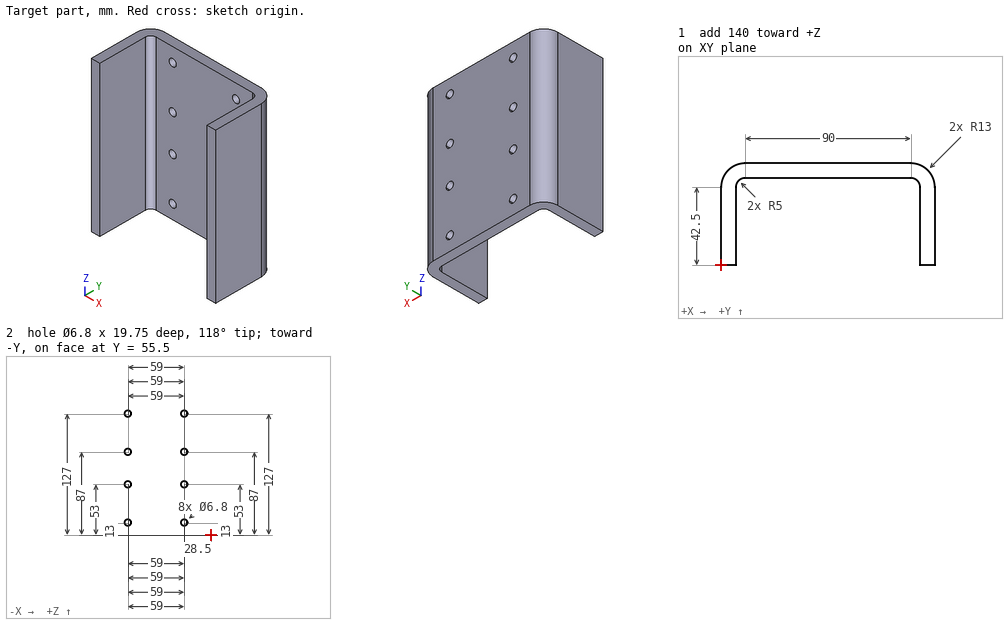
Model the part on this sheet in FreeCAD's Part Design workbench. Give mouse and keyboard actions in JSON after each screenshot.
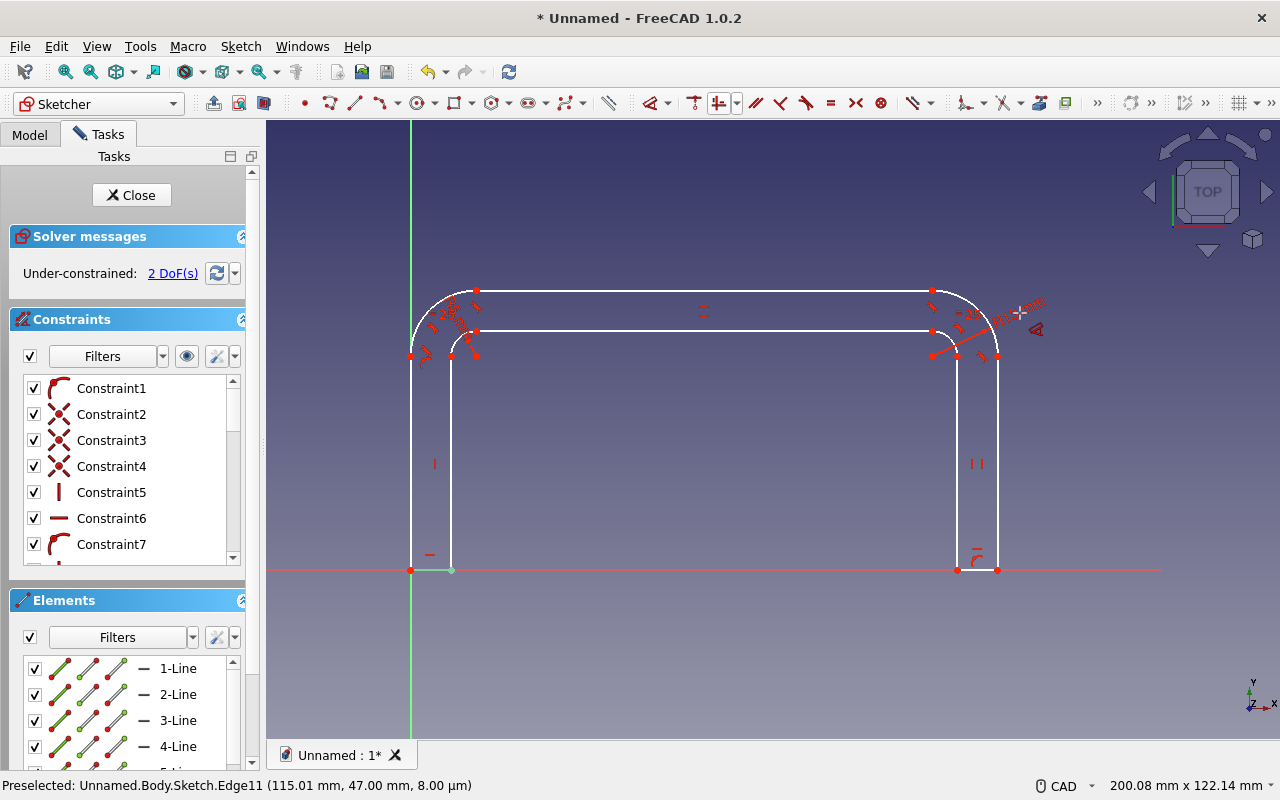
{"action": "left_click", "coordinate": [613, 331]}
{"action": "left_click", "coordinate": [704, 365]}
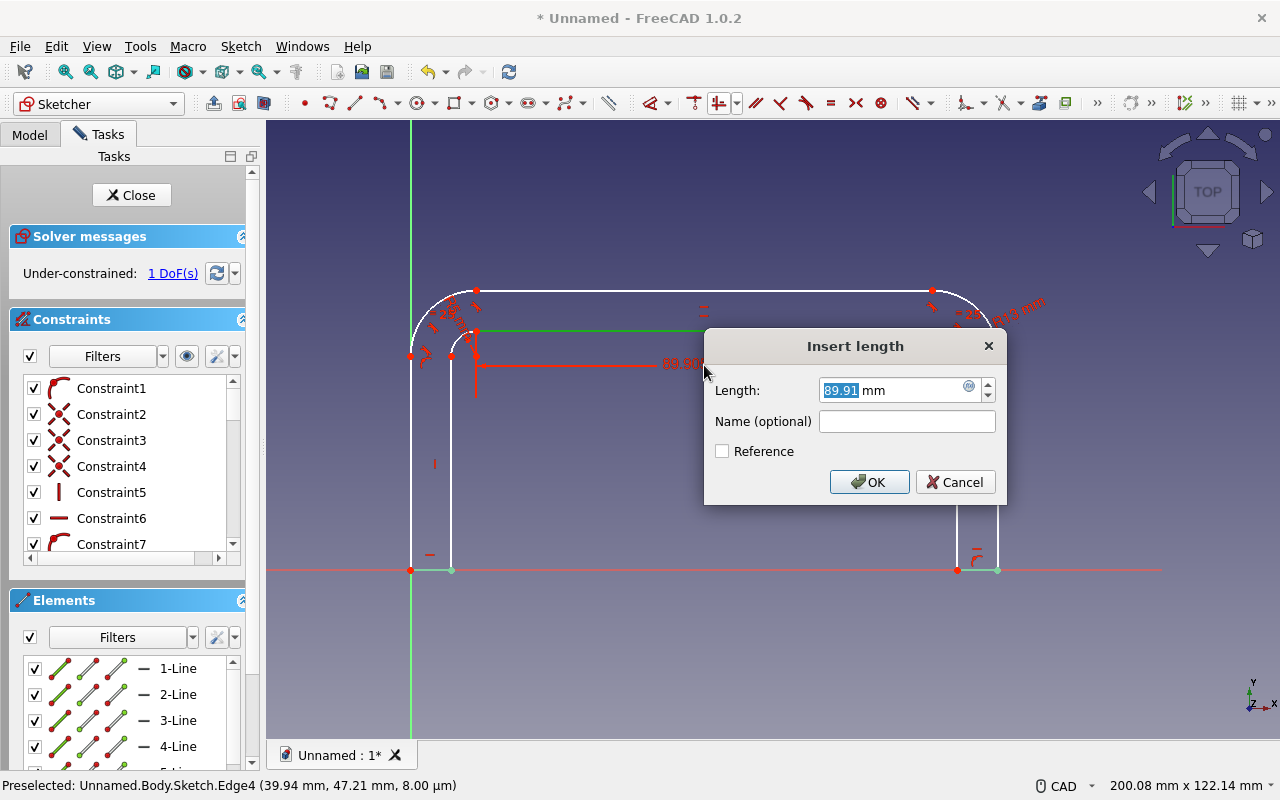
{"action": "type", "text": "90"}
{"action": "key", "text": "Return"}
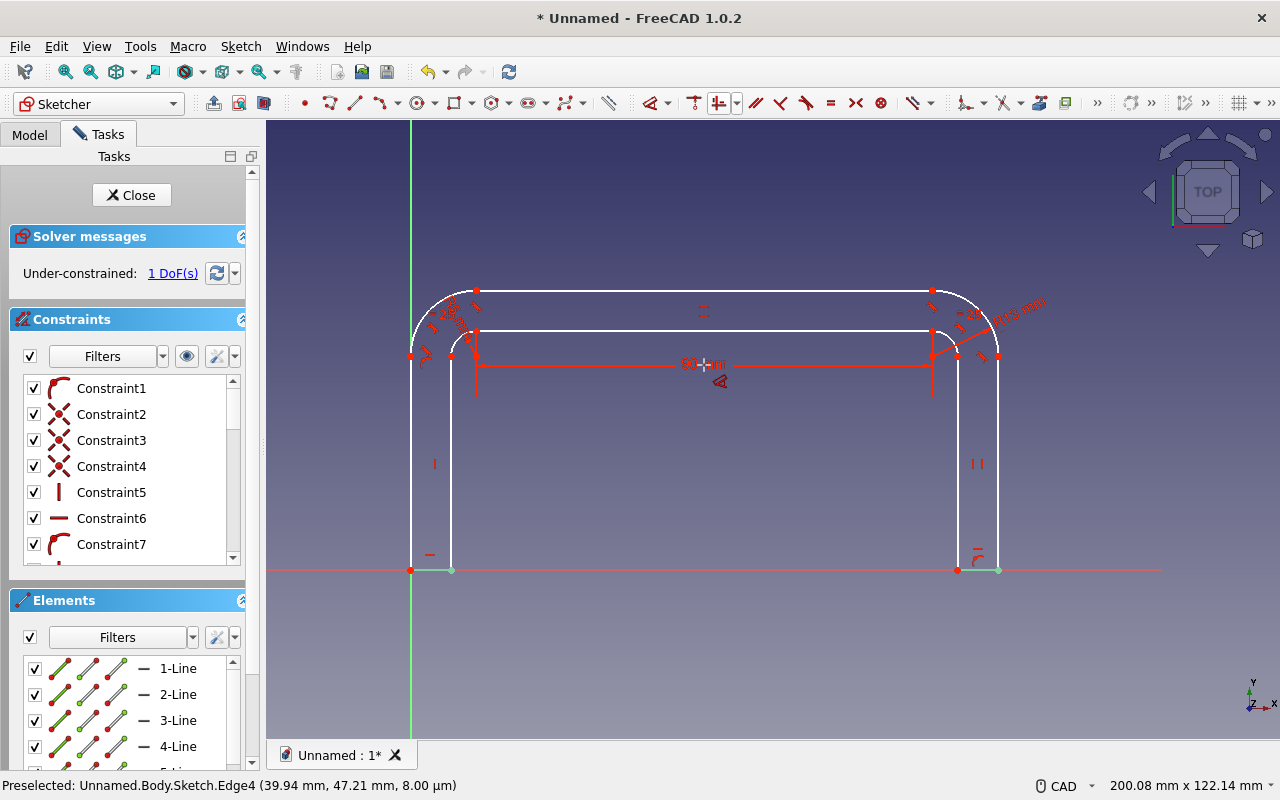
{"action": "left_click", "coordinate": [411, 421]}
{"action": "left_click", "coordinate": [377, 464]}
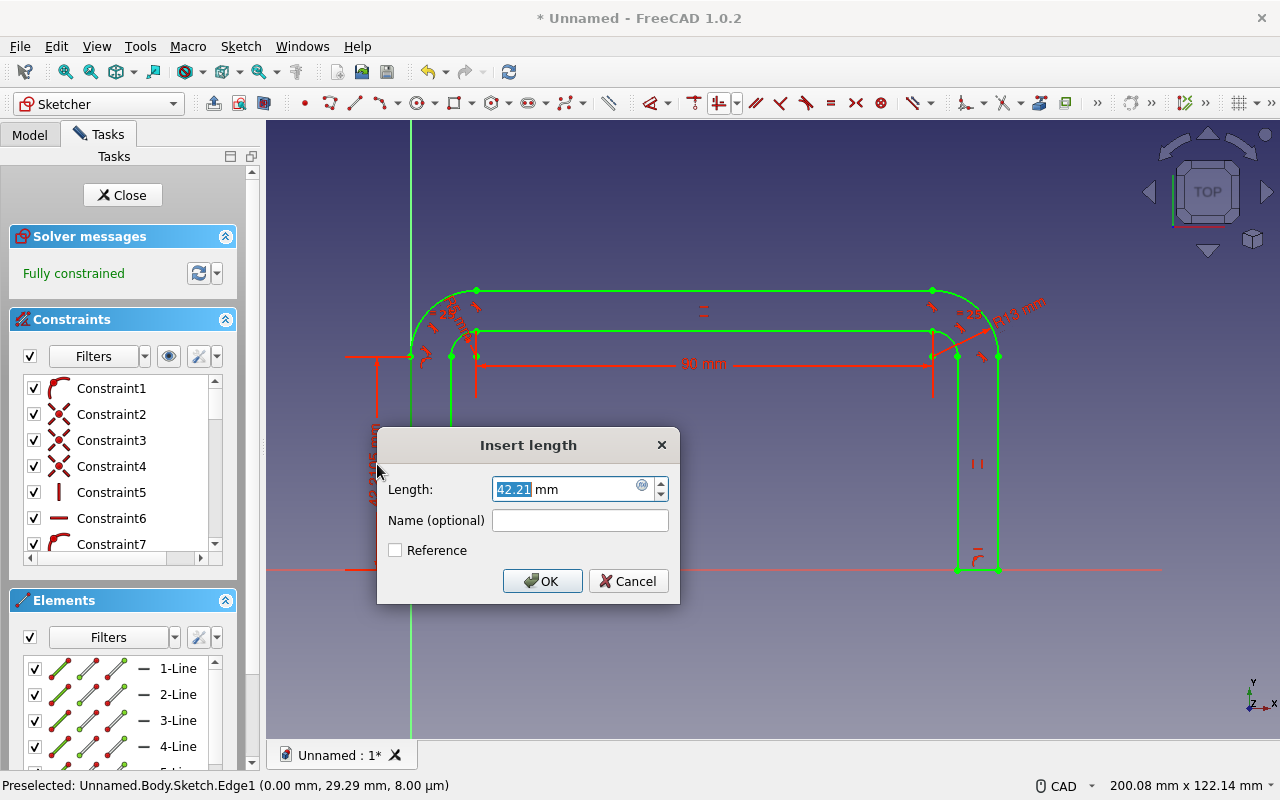
{"action": "type", "text": "42.5"}
{"action": "key", "text": "Return"}
{"action": "key", "text": "Escape"}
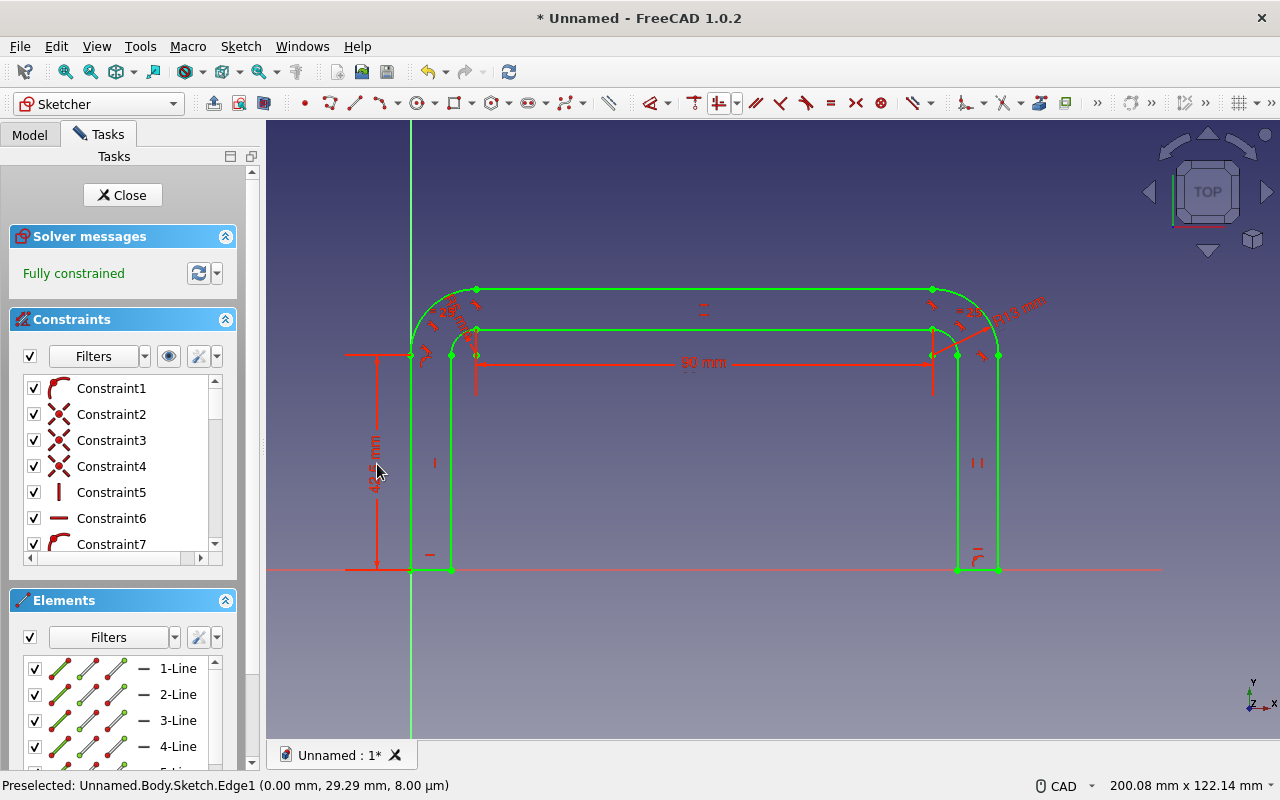
{"action": "left_click", "coordinate": [123, 195]}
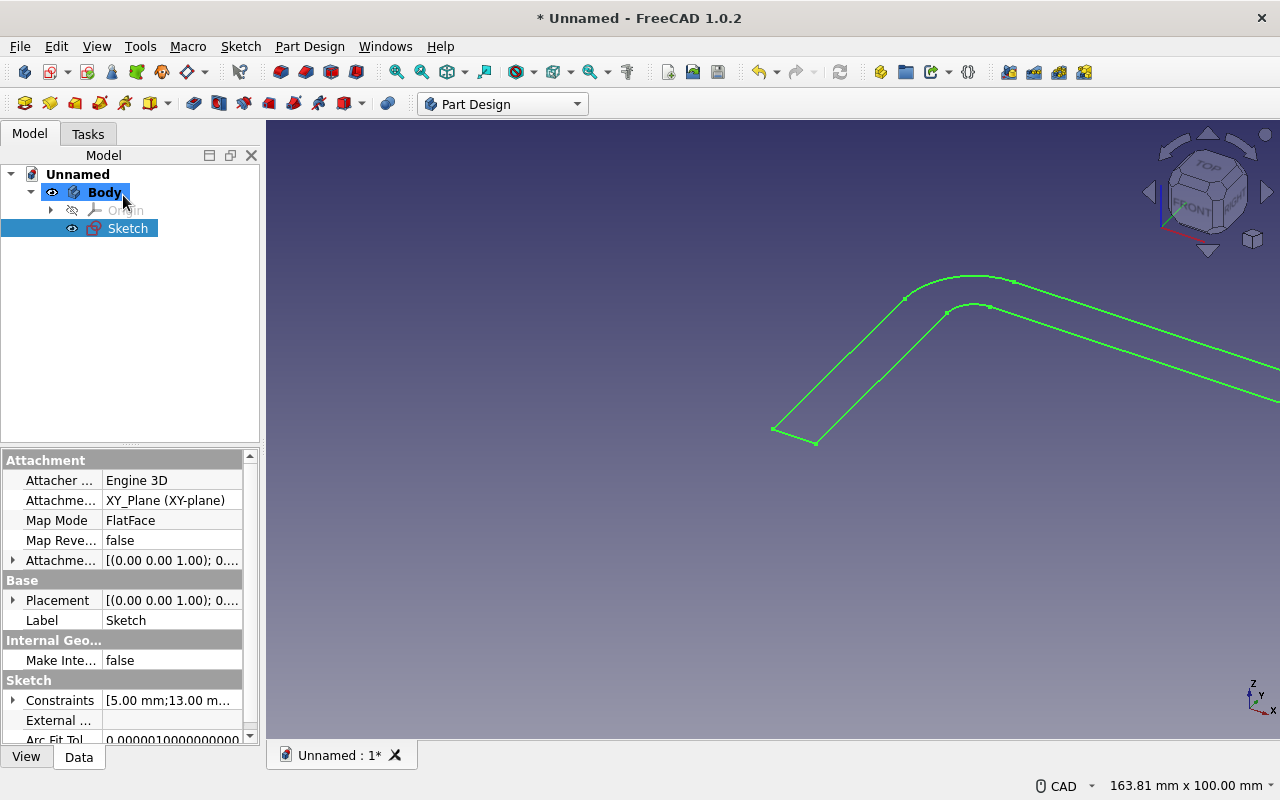
{"action": "left_click", "coordinate": [25, 104]}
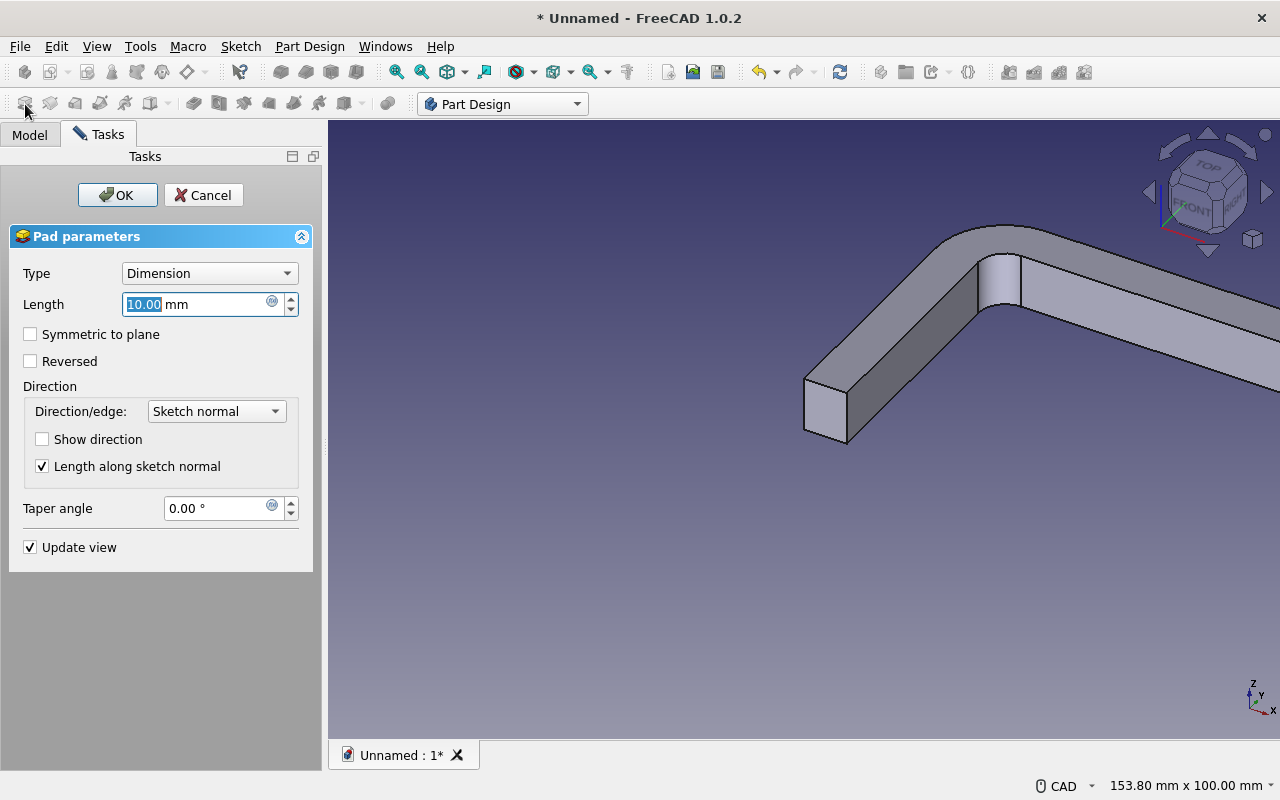
{"action": "type", "text": "140"}
{"action": "key", "text": "Tab"}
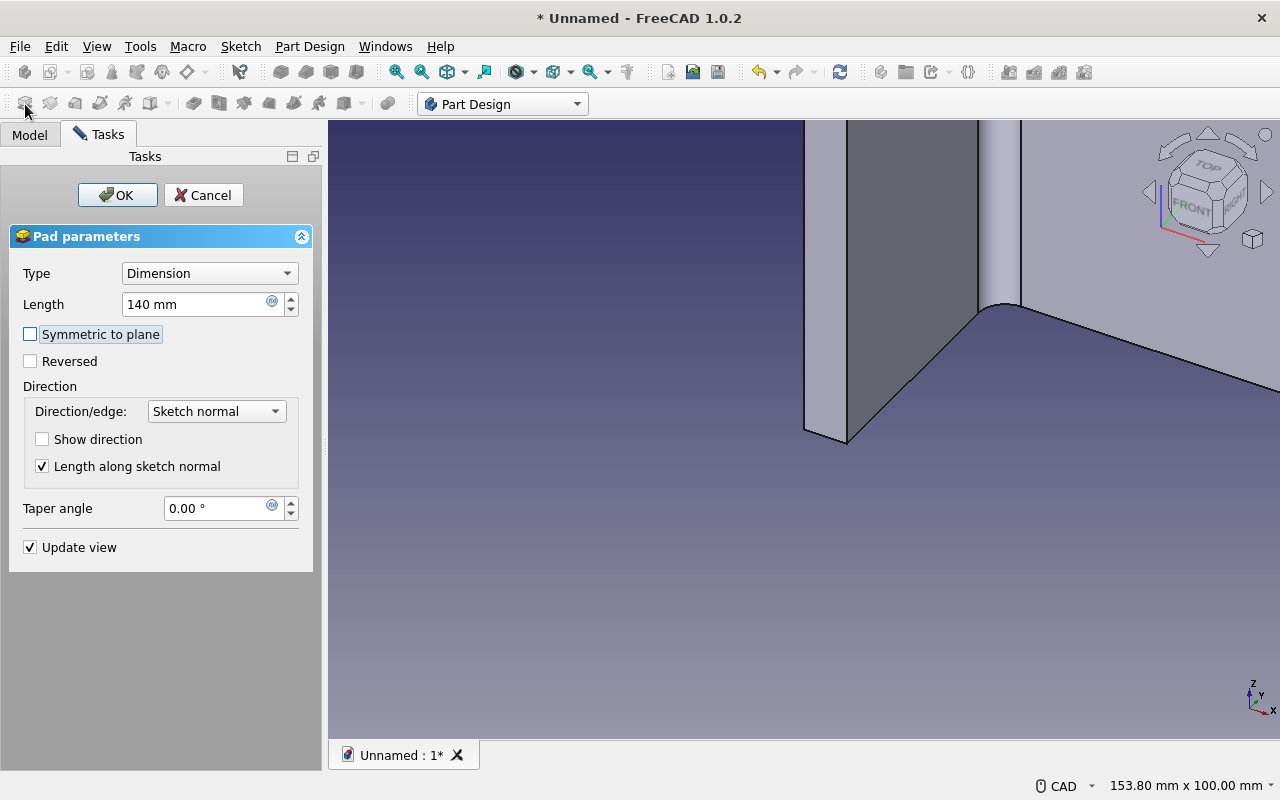
{"action": "left_click", "coordinate": [118, 195]}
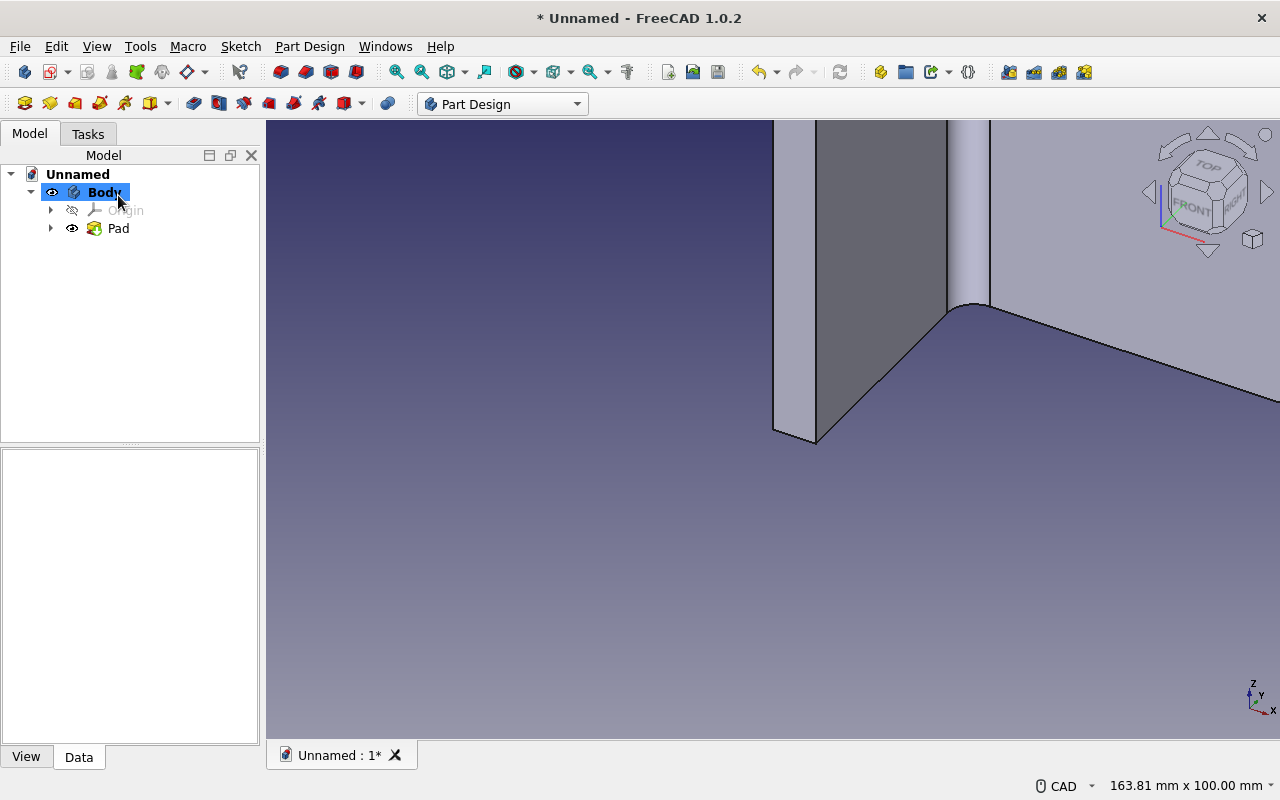
{"action": "left_click", "coordinate": [397, 72]}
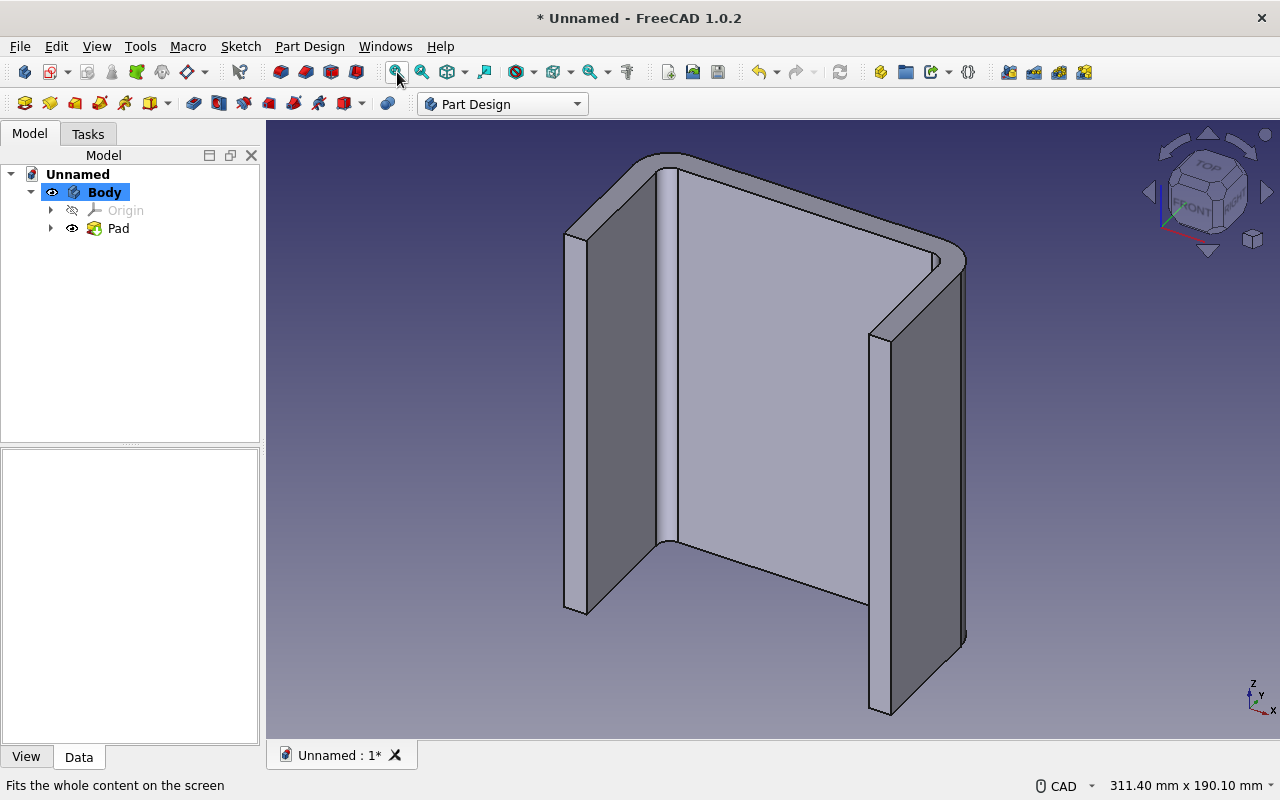
{"action": "key", "text": "4"}